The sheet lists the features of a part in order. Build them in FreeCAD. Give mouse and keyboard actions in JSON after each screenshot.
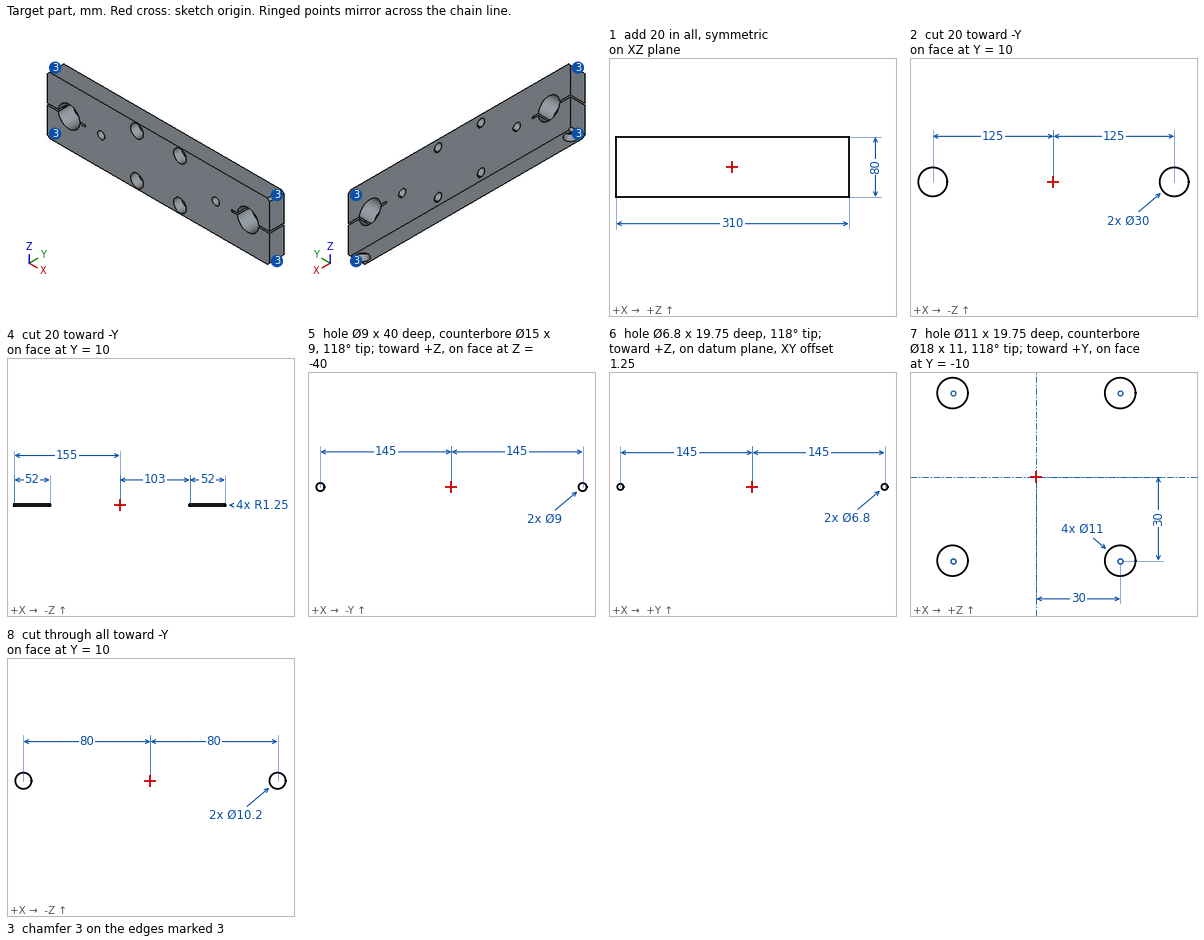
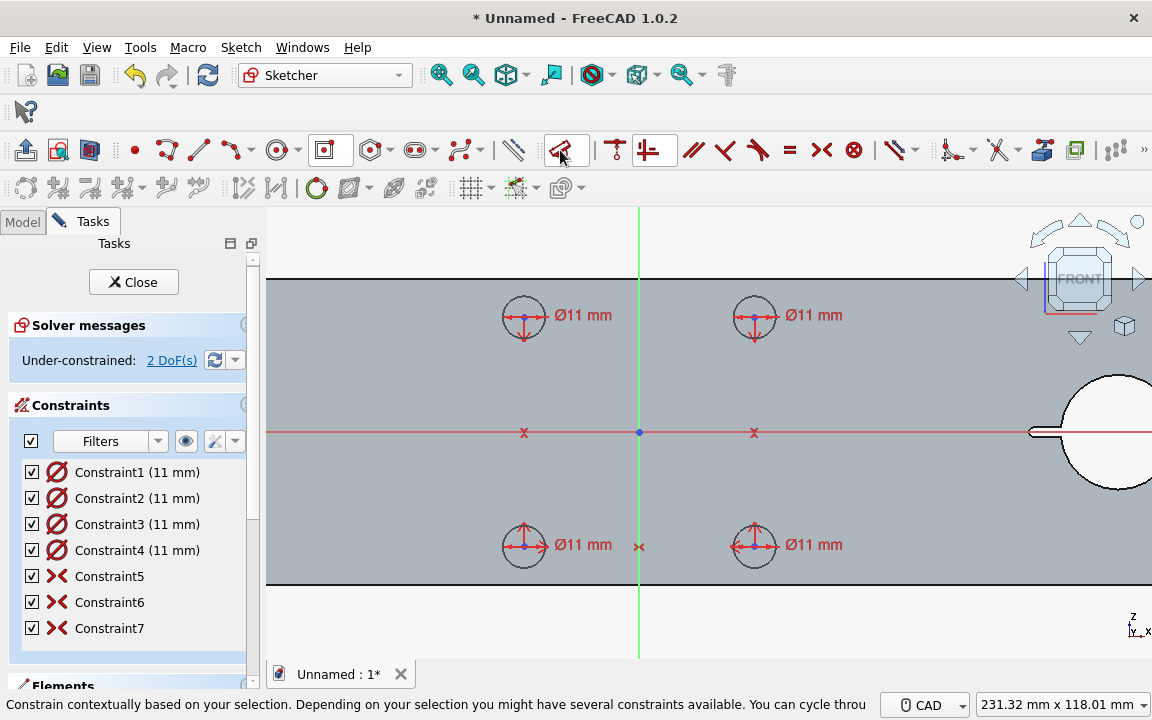
{"action": "left_click", "coordinate": [755, 547]}
{"action": "left_click", "coordinate": [697, 581]}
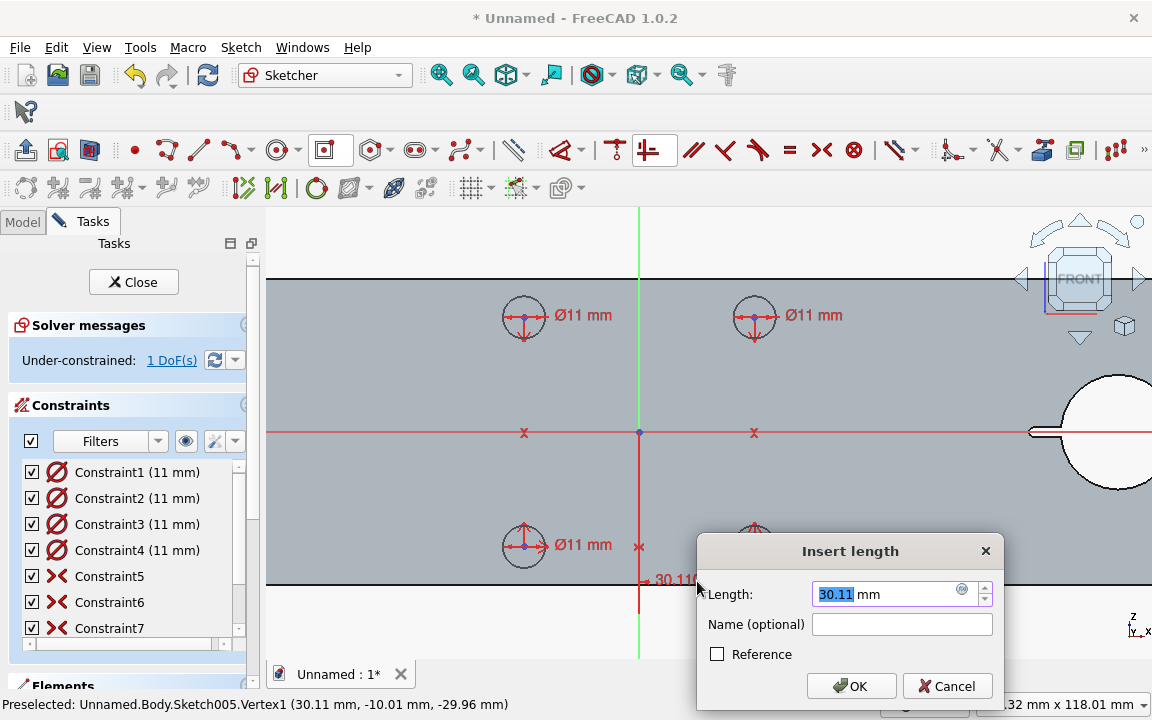
{"action": "type", "text": "30"}
{"action": "key", "text": "Return"}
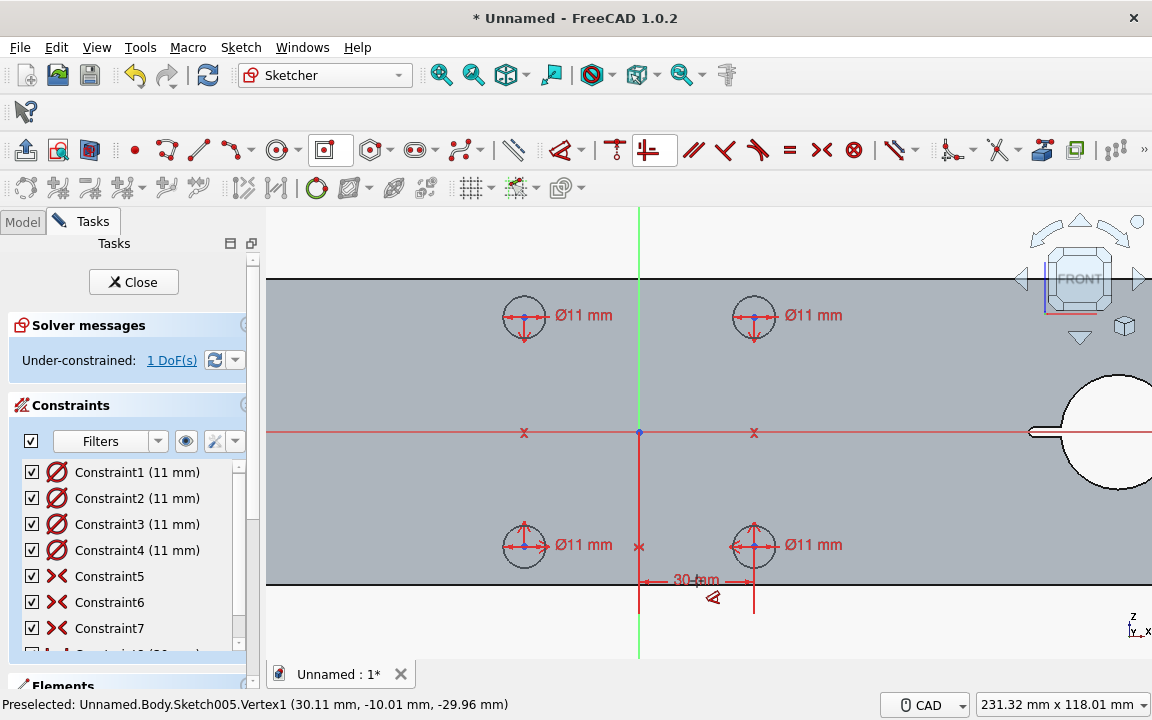
{"action": "left_click", "coordinate": [754, 547]}
{"action": "left_click", "coordinate": [788, 490]}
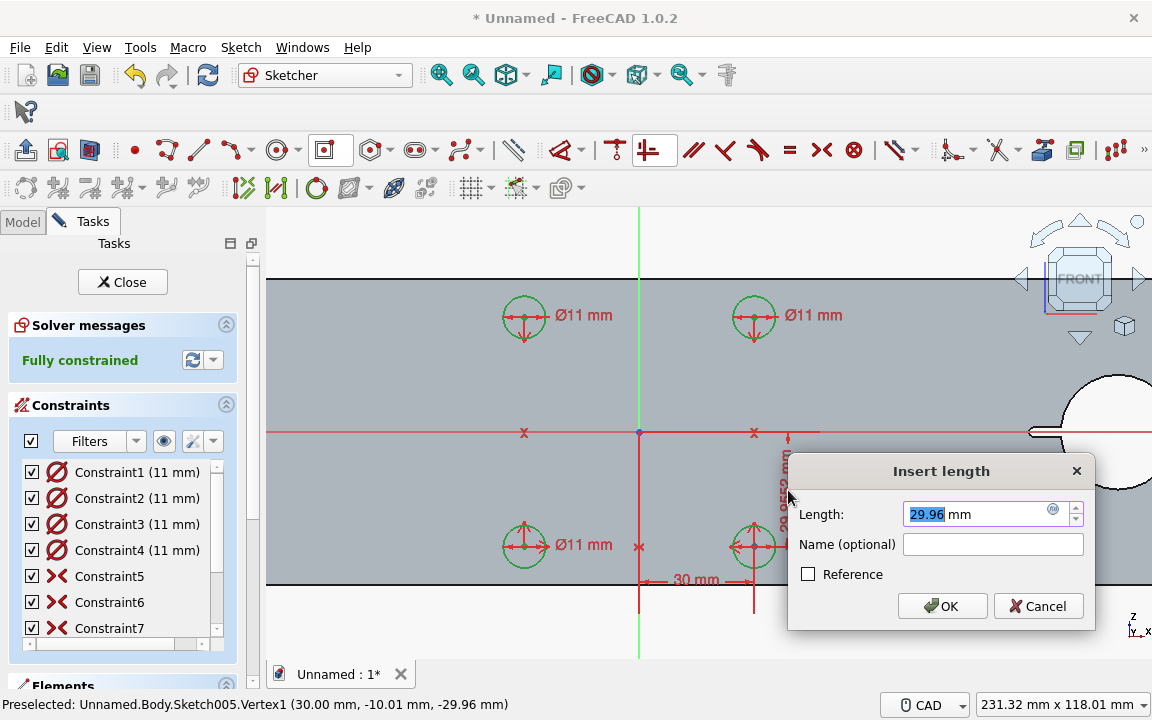
{"action": "type", "text": "30"}
{"action": "key", "text": "Return"}
{"action": "key", "text": "Escape"}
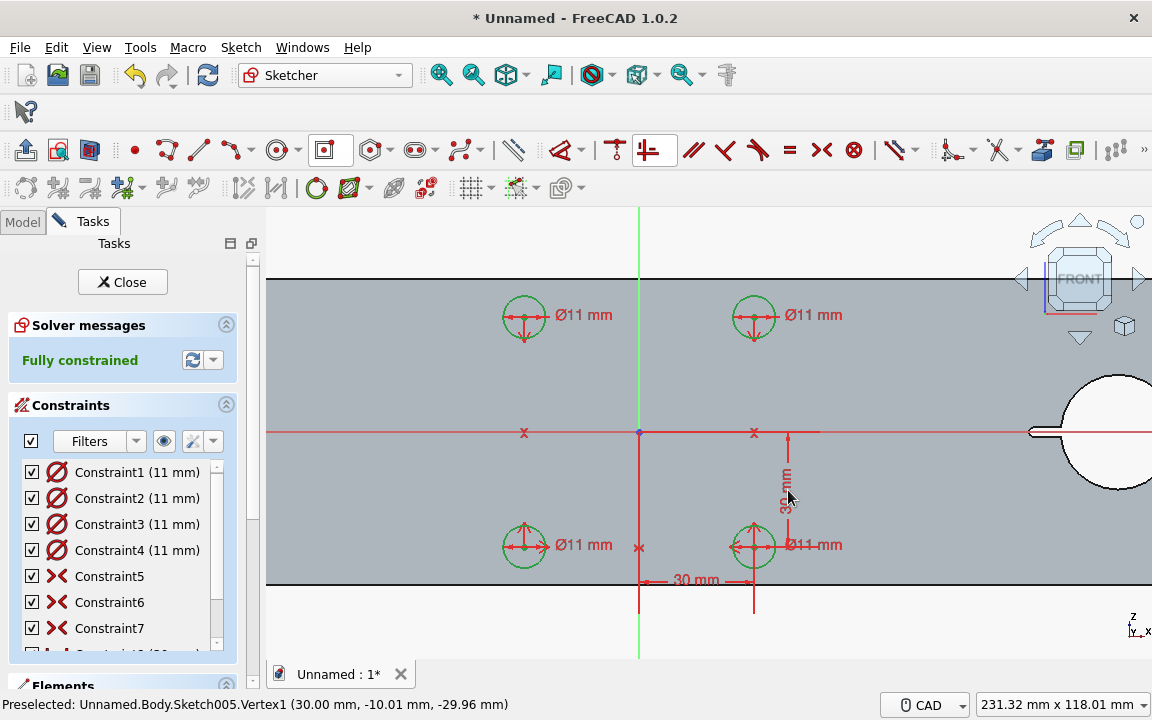
{"action": "left_click", "coordinate": [123, 282]}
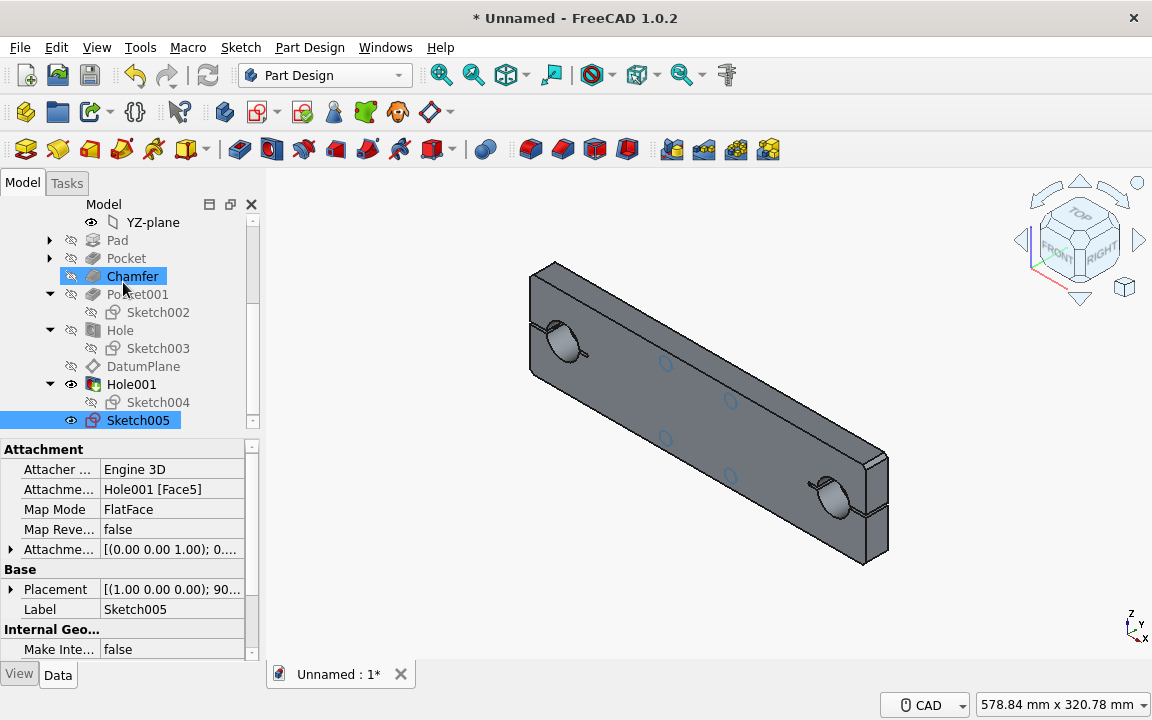
{"action": "left_click", "coordinate": [272, 150]}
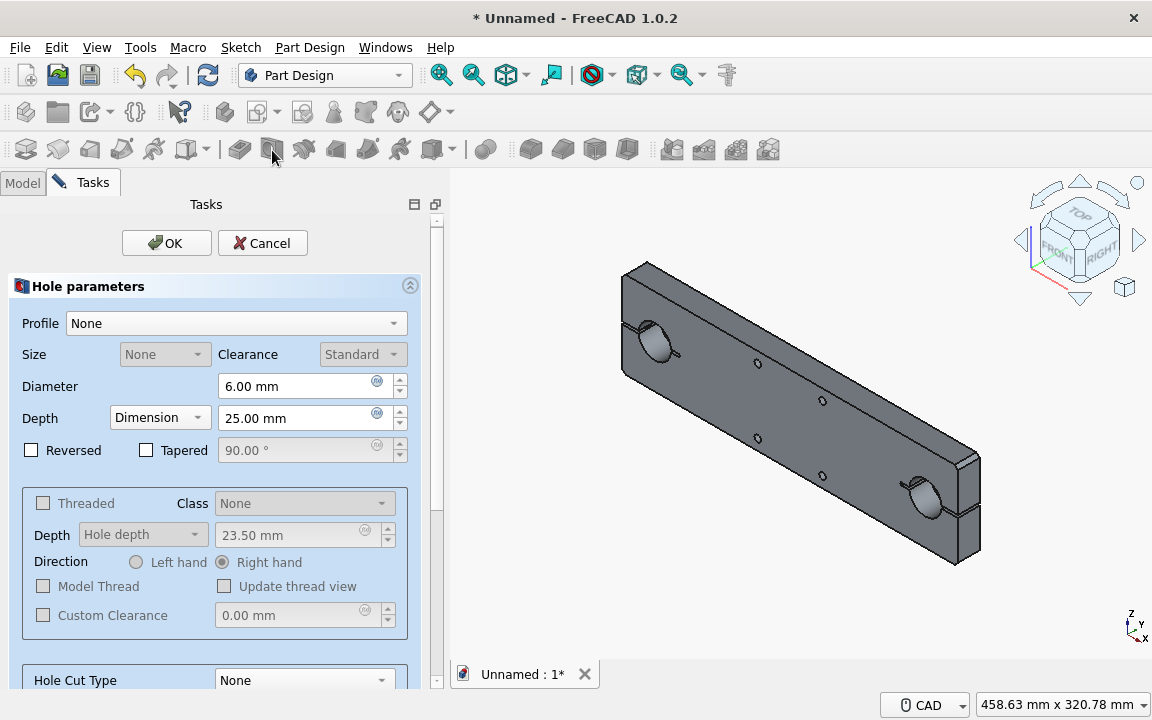
{"action": "triple_click", "coordinate": [305, 386]}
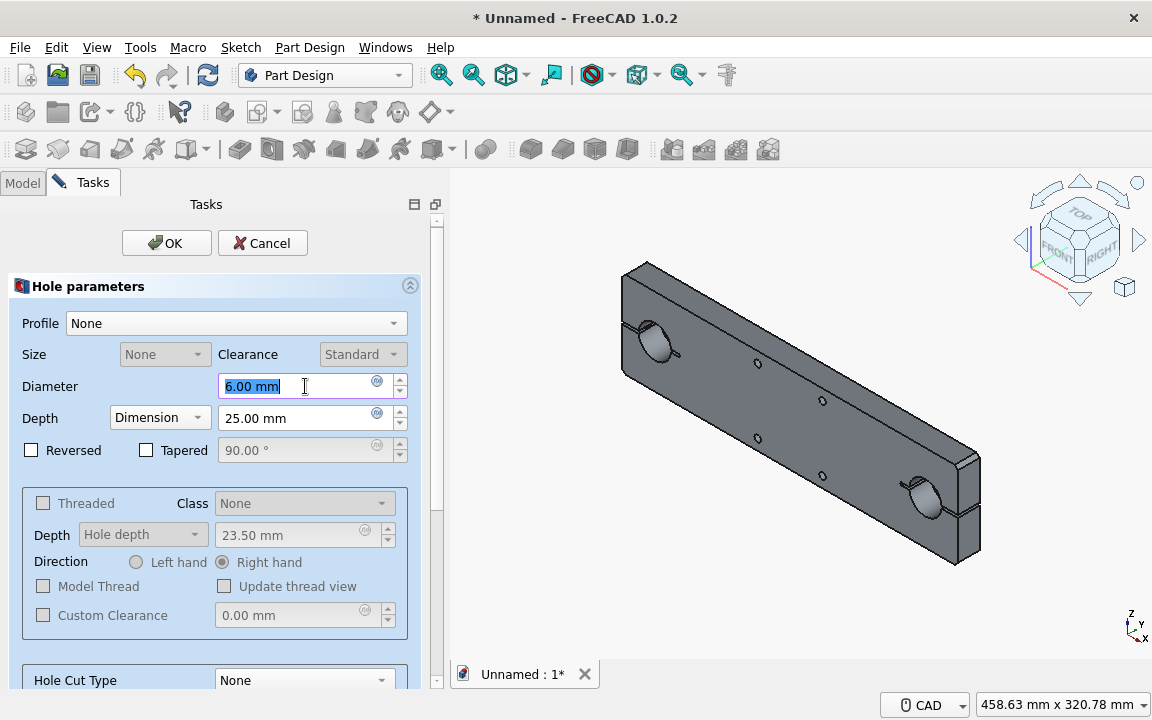
{"action": "type", "text": "11"}
{"action": "key", "text": "Tab"}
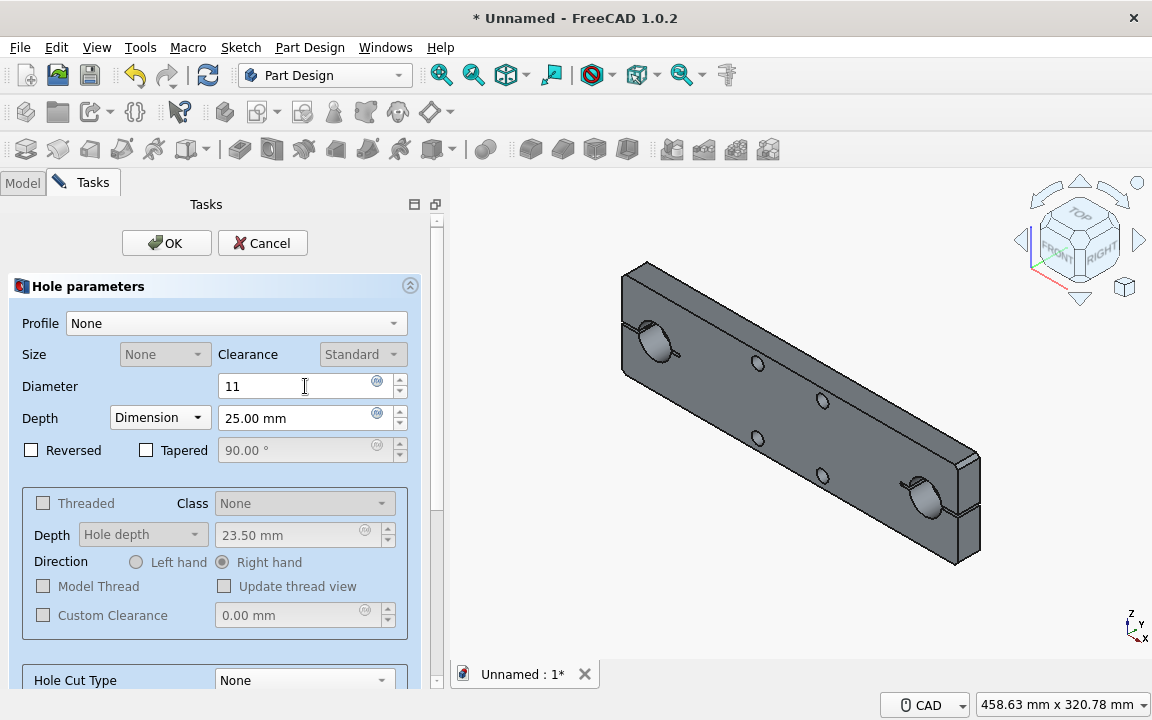
{"action": "triple_click", "coordinate": [305, 418]}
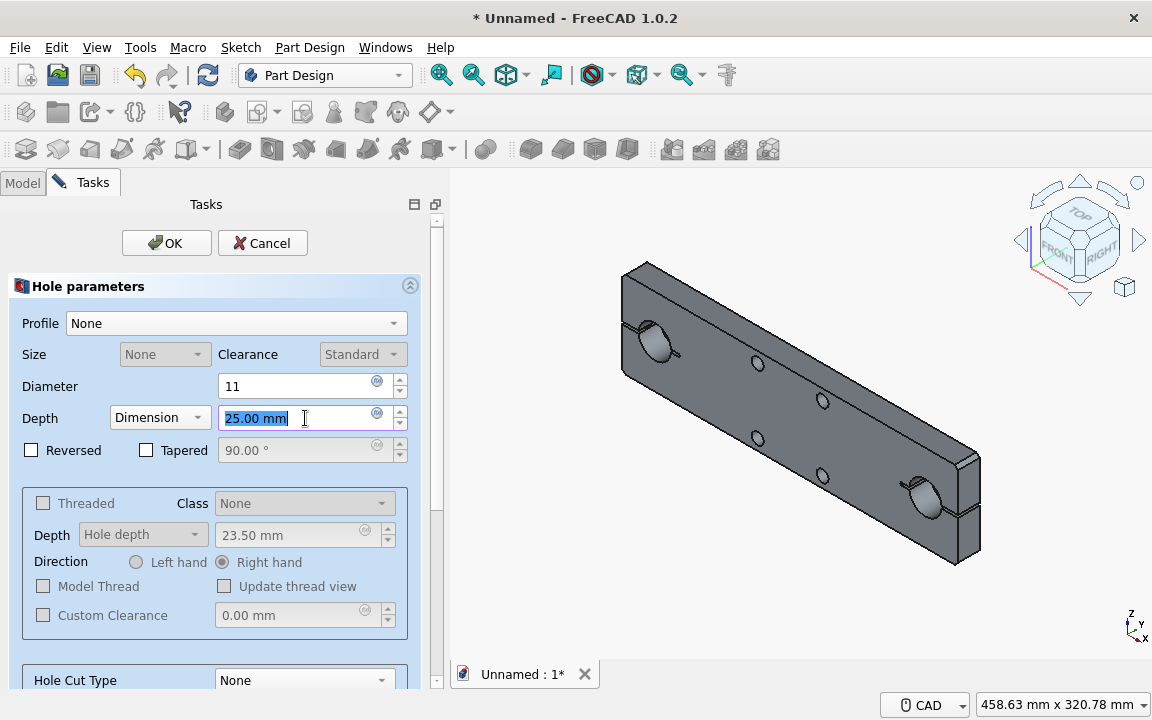
{"action": "type", "text": "19.75"}
{"action": "key", "text": "Tab"}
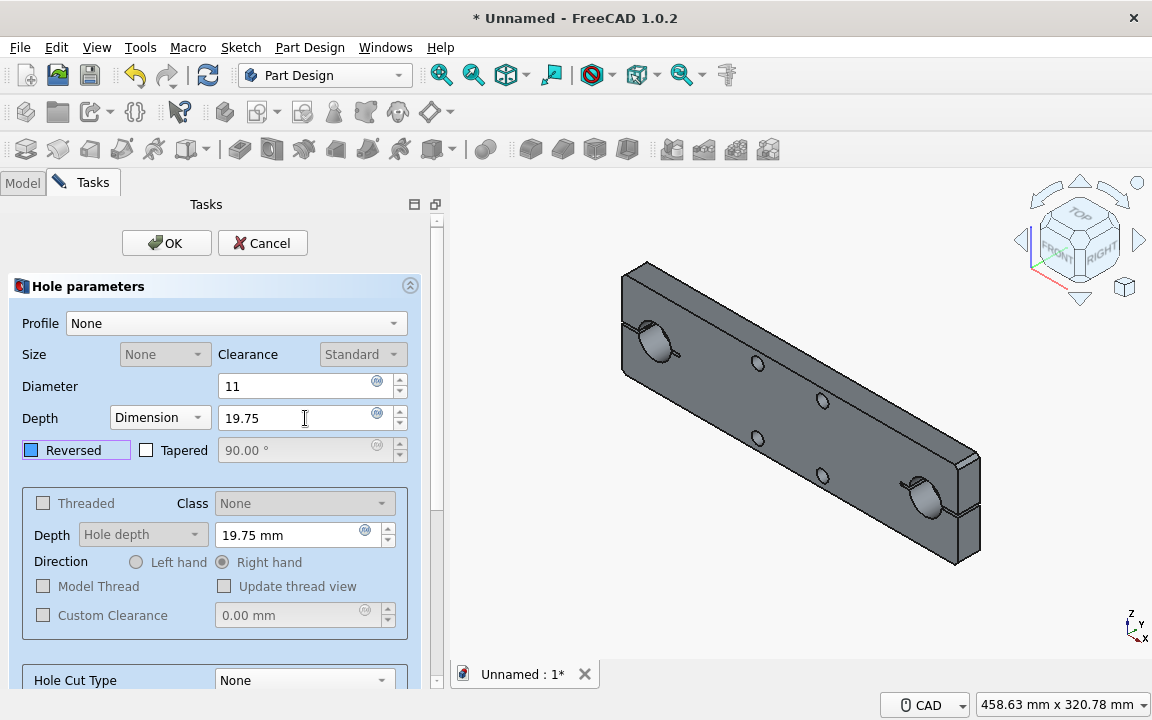
{"action": "scroll", "coordinate": [437, 451], "scroll_direction": "down", "scroll_amount": 2}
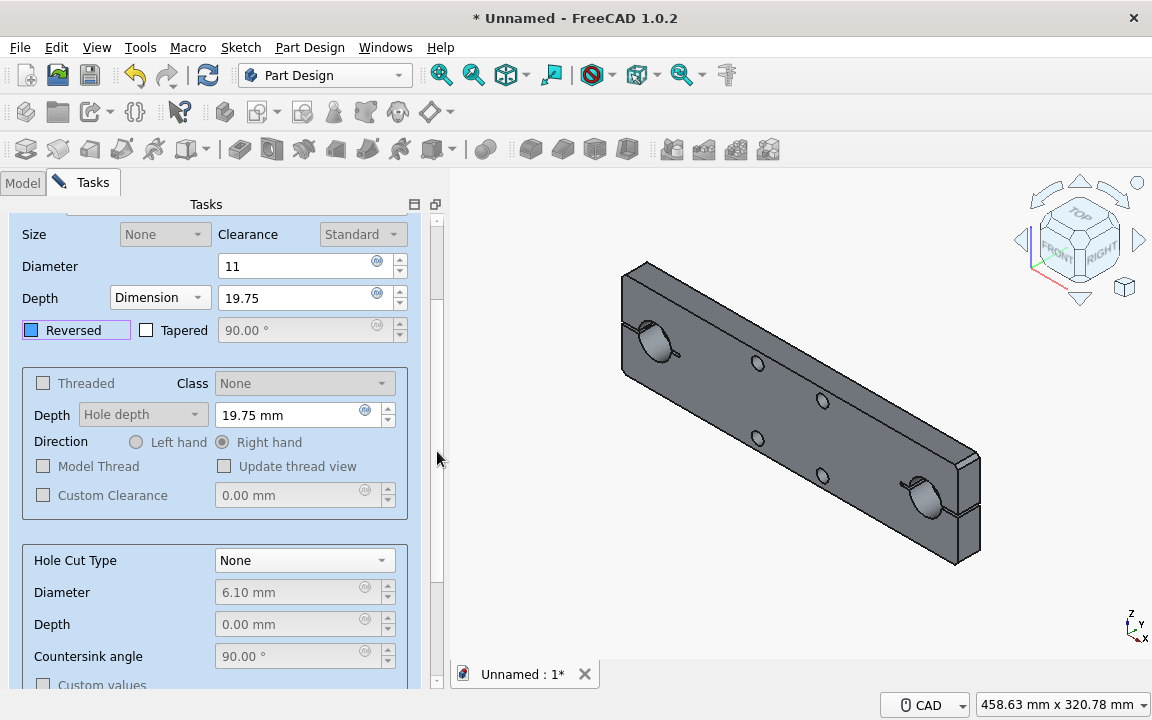
{"action": "left_click", "coordinate": [306, 560]}